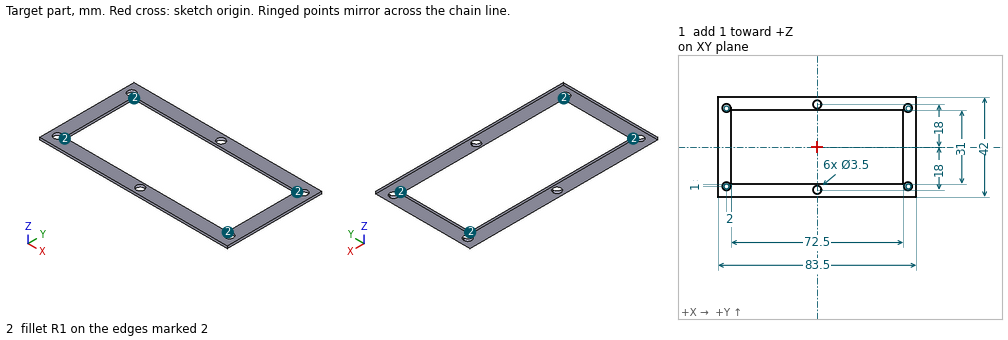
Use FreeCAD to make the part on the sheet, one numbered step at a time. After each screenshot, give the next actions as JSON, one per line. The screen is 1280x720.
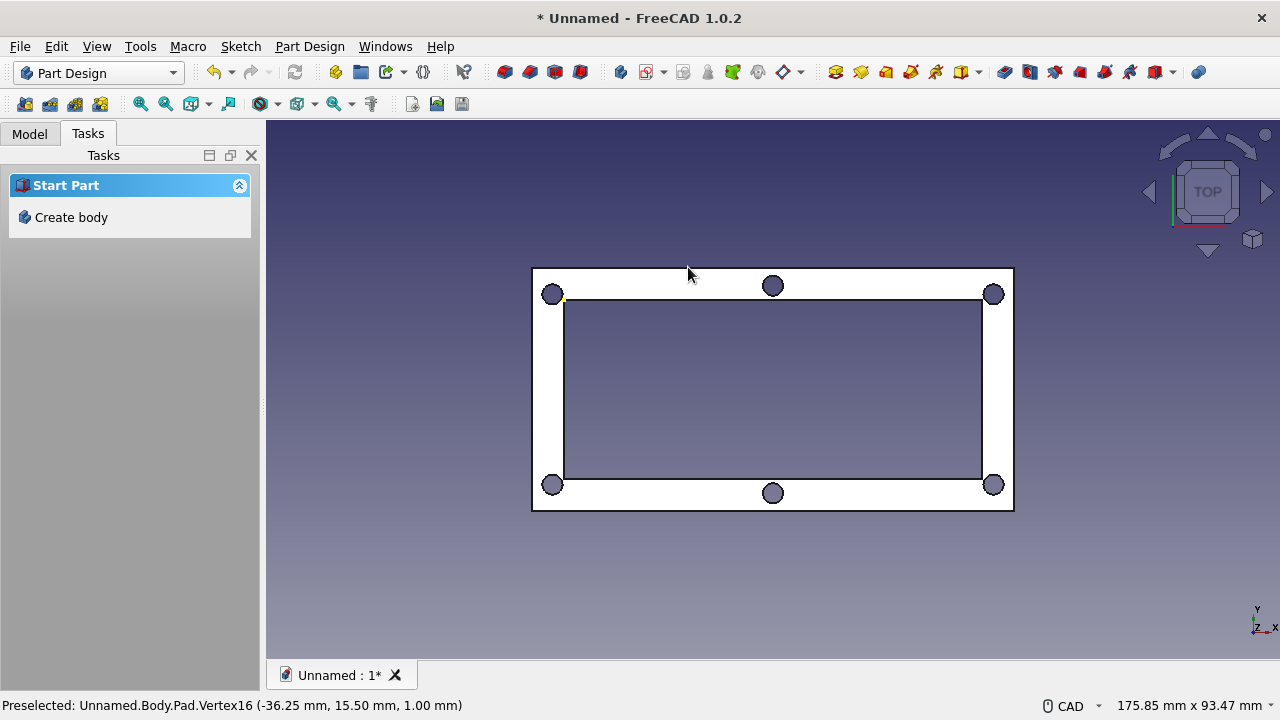
{"action": "scroll", "coordinate": [564, 299], "scroll_direction": "up", "scroll_amount": 10}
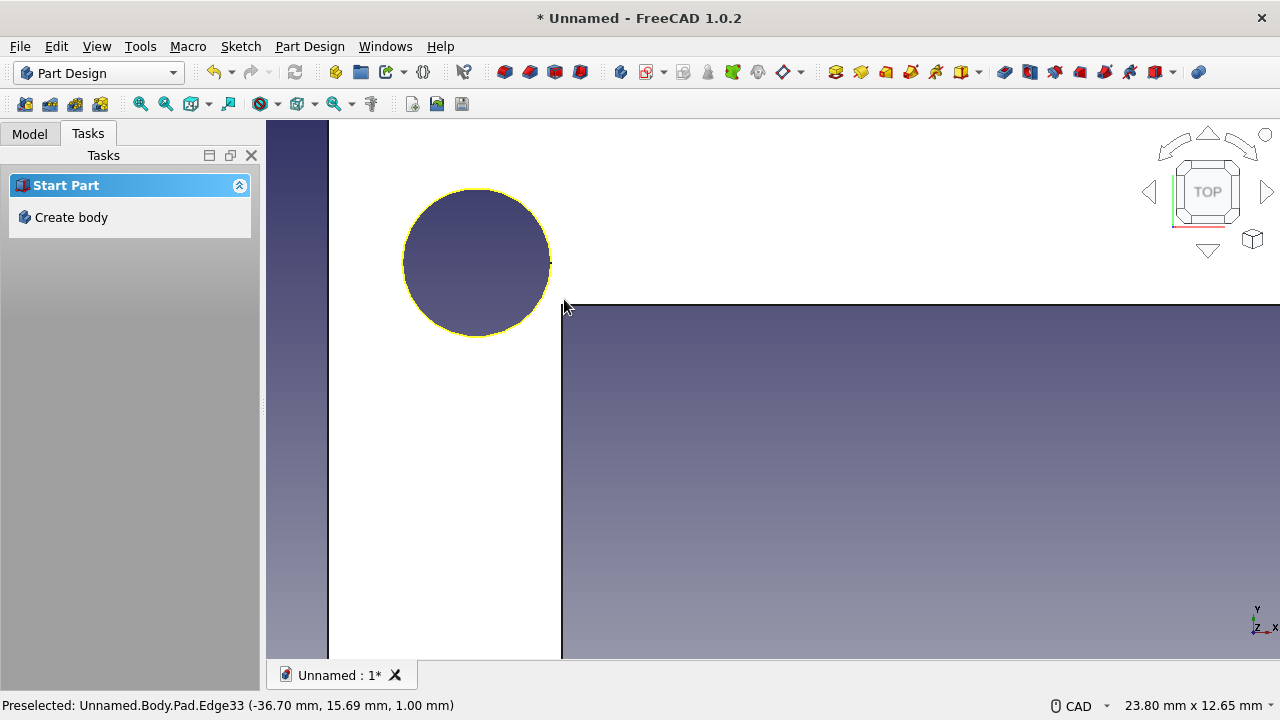
{"action": "key", "text": "v f"}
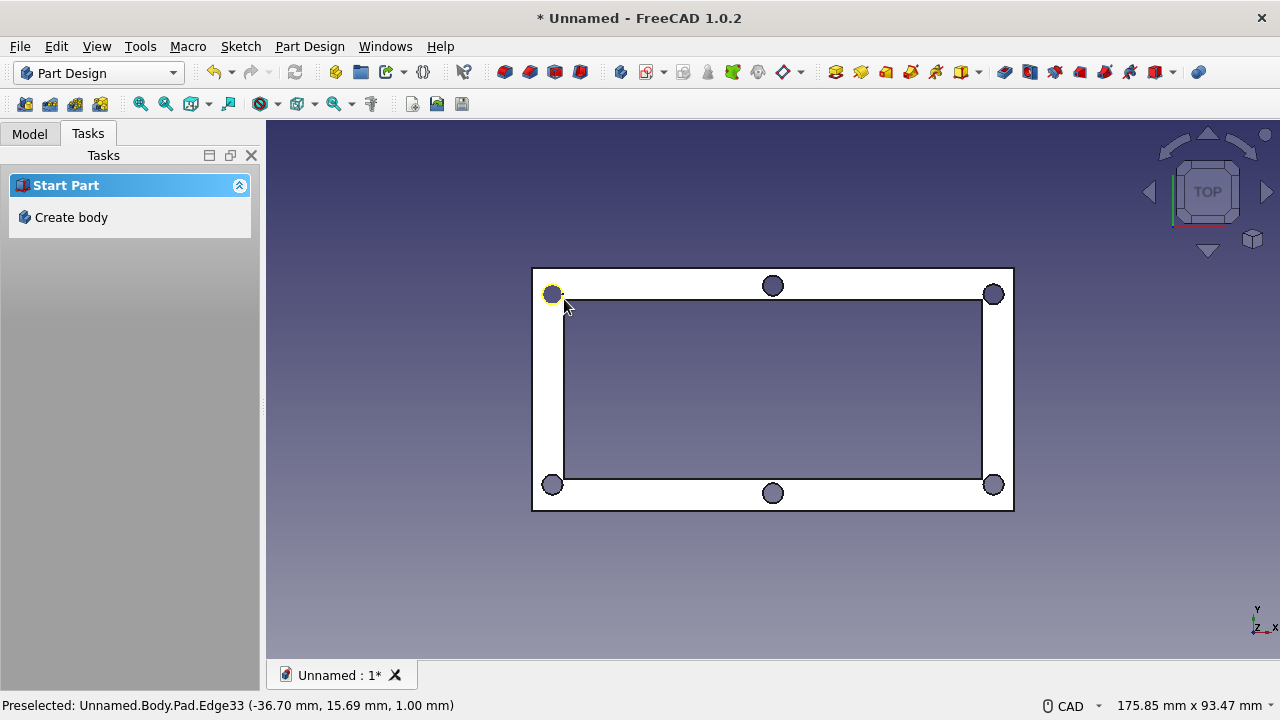
{"action": "key", "text": "1"}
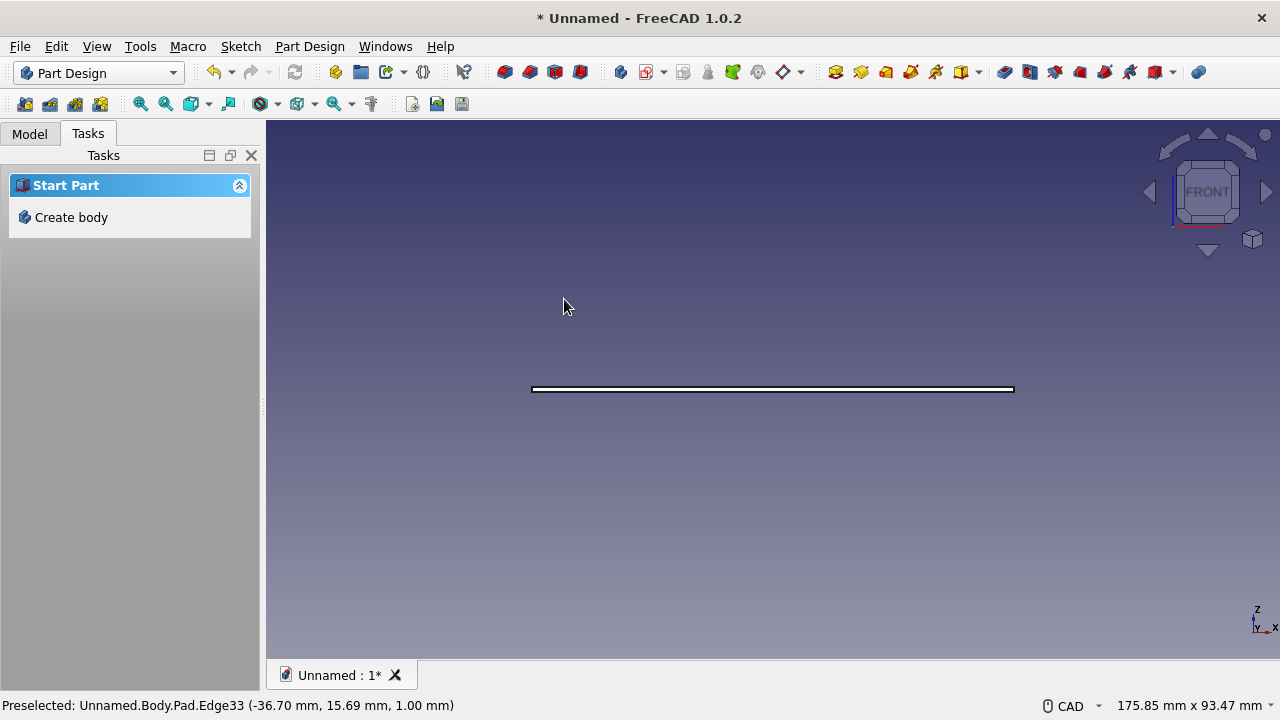
{"action": "scroll", "coordinate": [564, 389], "scroll_direction": "up", "scroll_amount": 10}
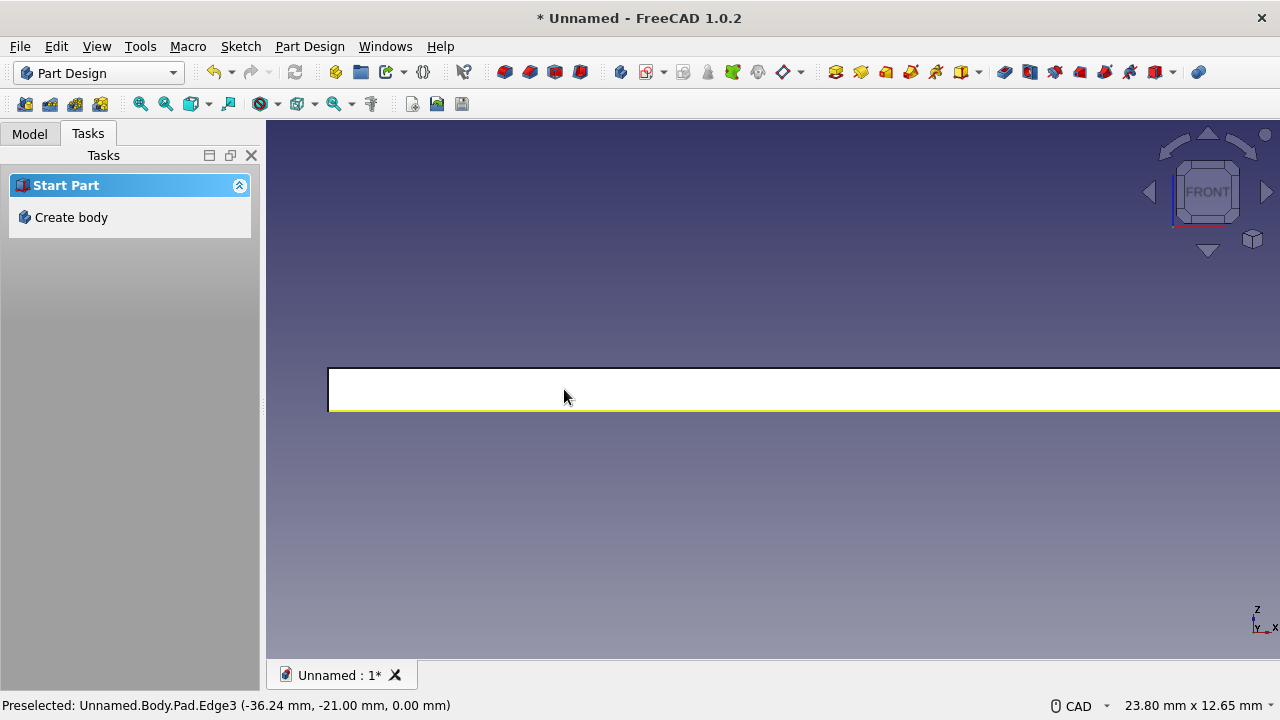
{"action": "key", "text": "v f"}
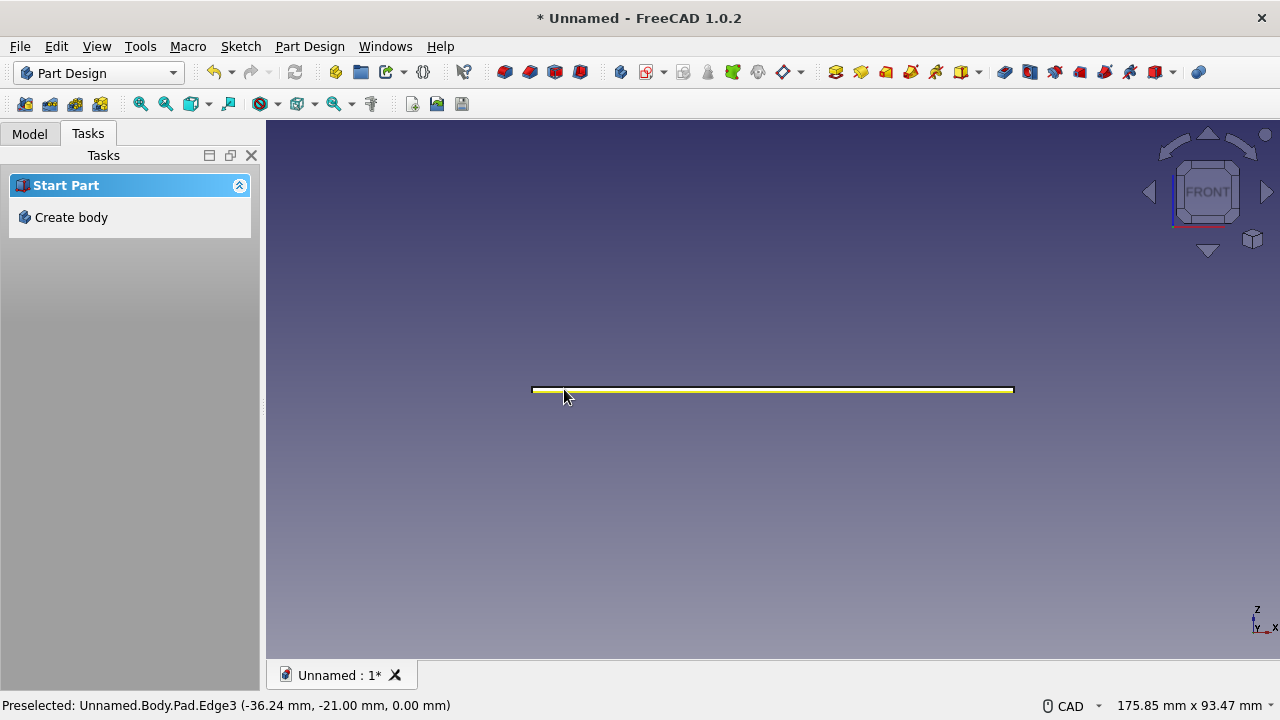
{"action": "key", "text": "3"}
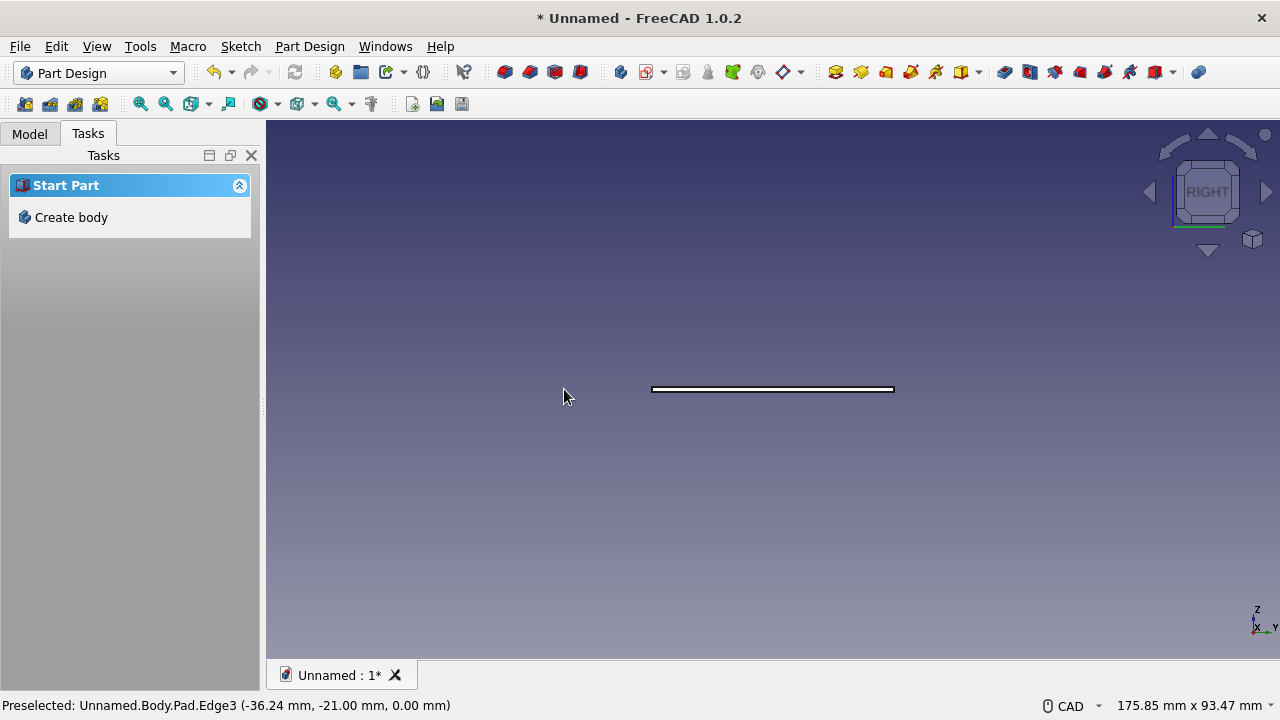
{"action": "key", "text": "v f"}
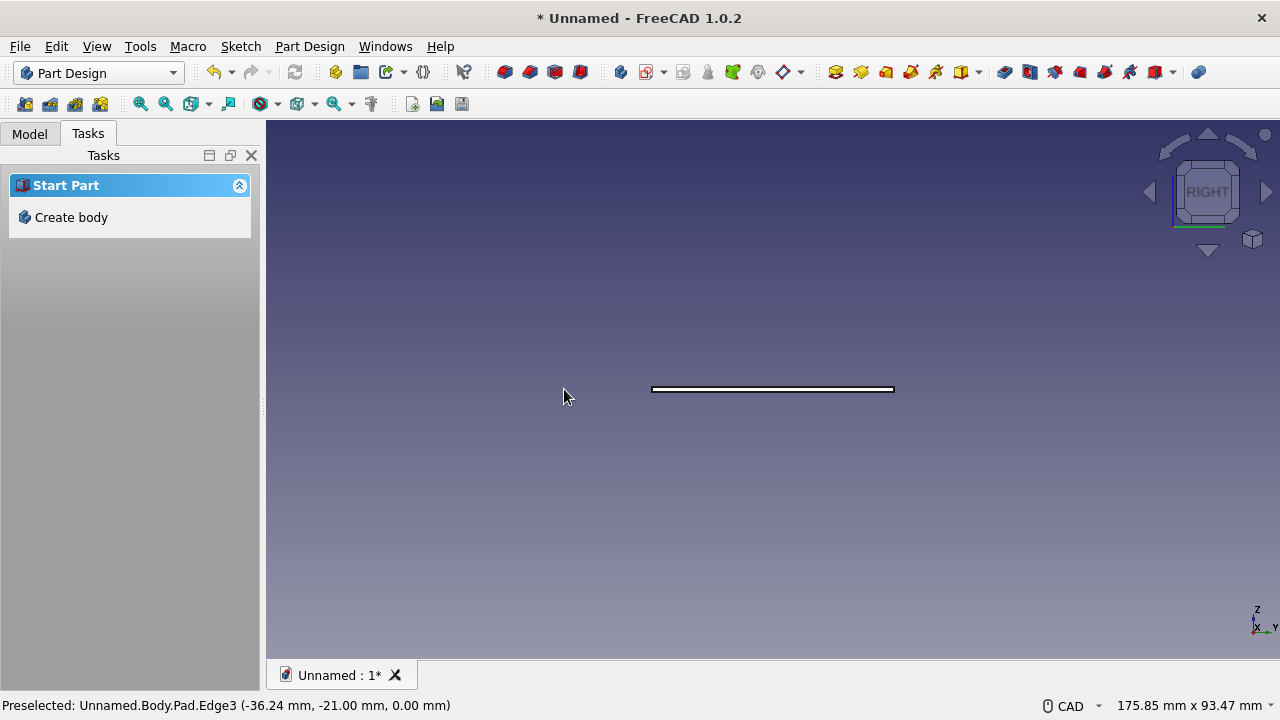
{"action": "scroll", "coordinate": [862, 388], "scroll_direction": "up", "scroll_amount": 10}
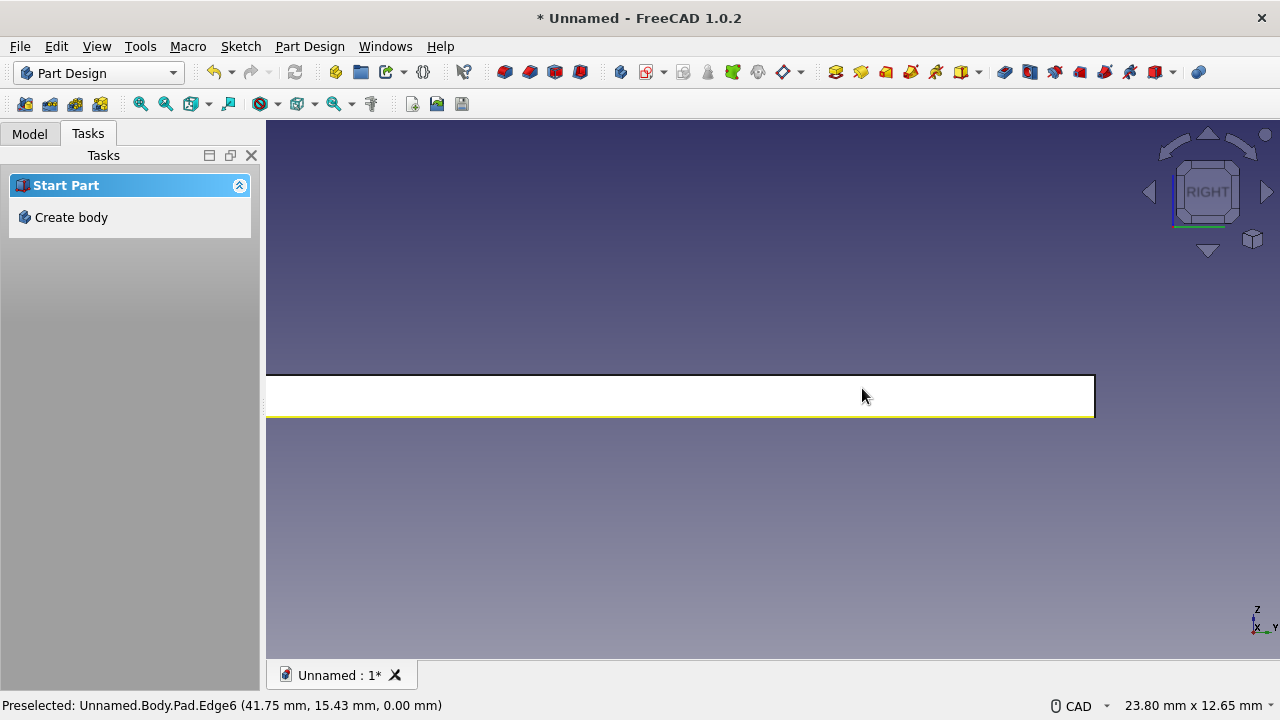
{"action": "key", "text": "v f"}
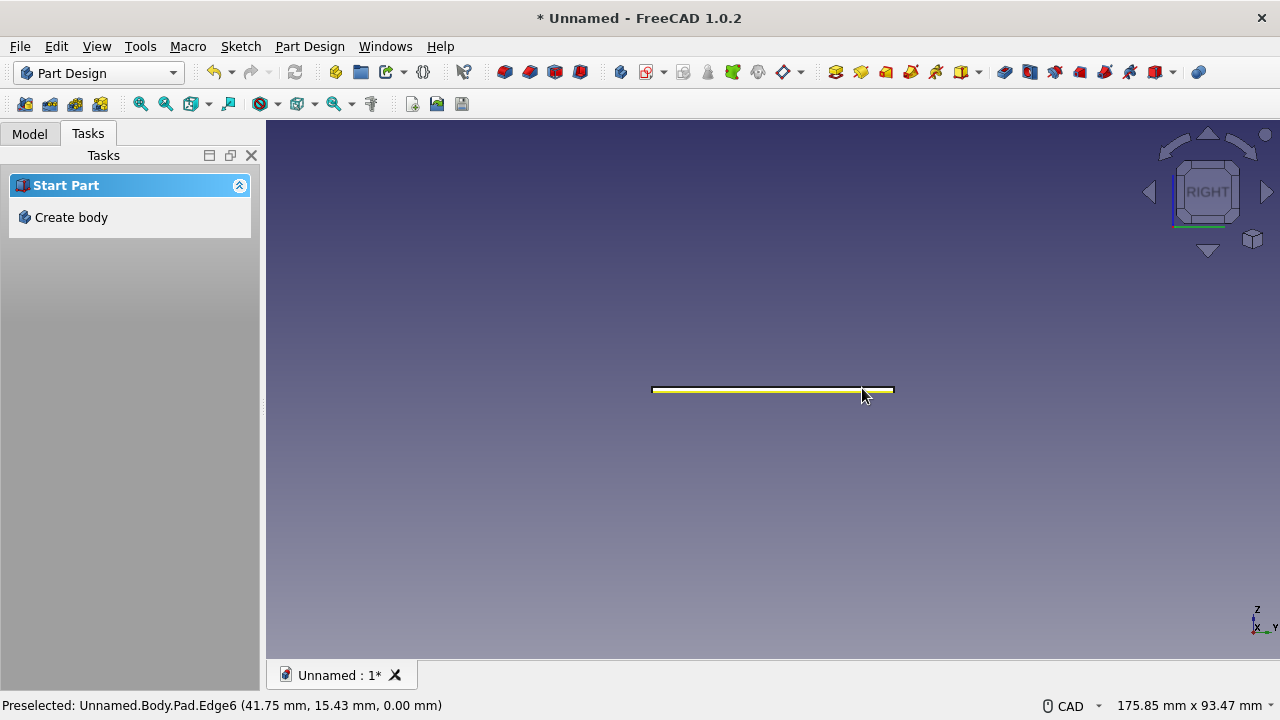
{"action": "key", "text": "5"}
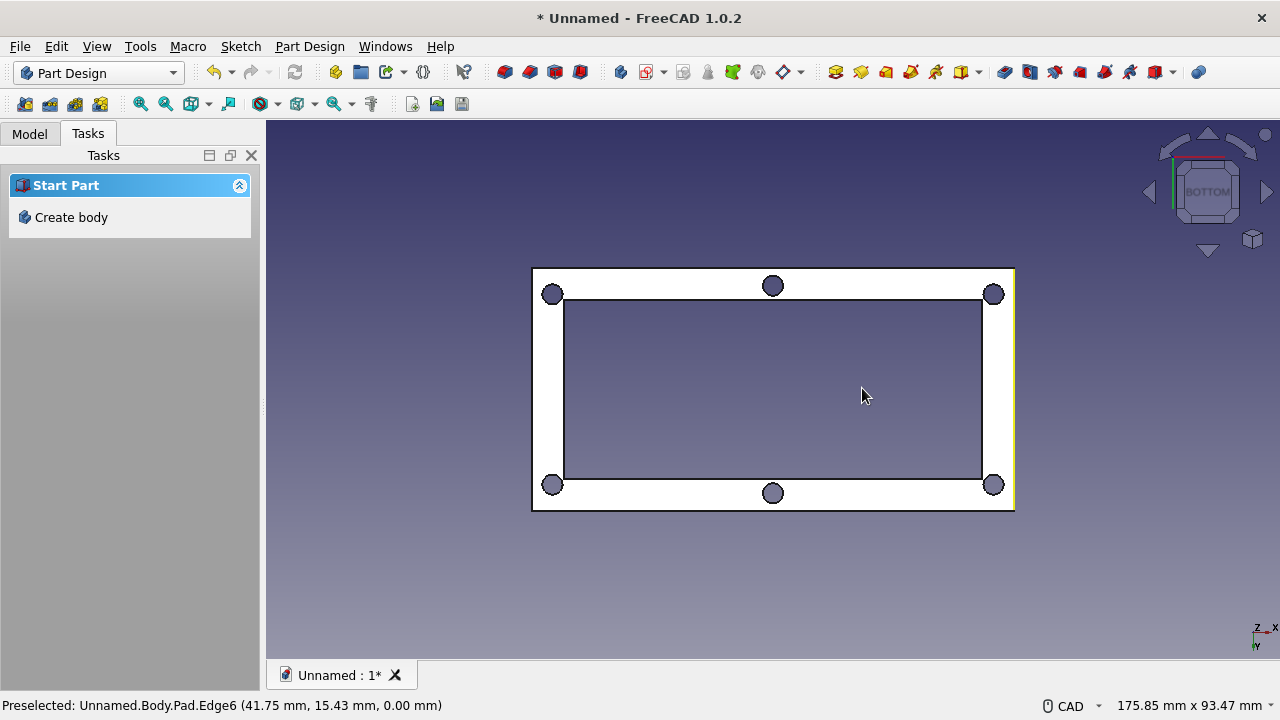
{"action": "scroll", "coordinate": [564, 478], "scroll_direction": "up", "scroll_amount": 10}